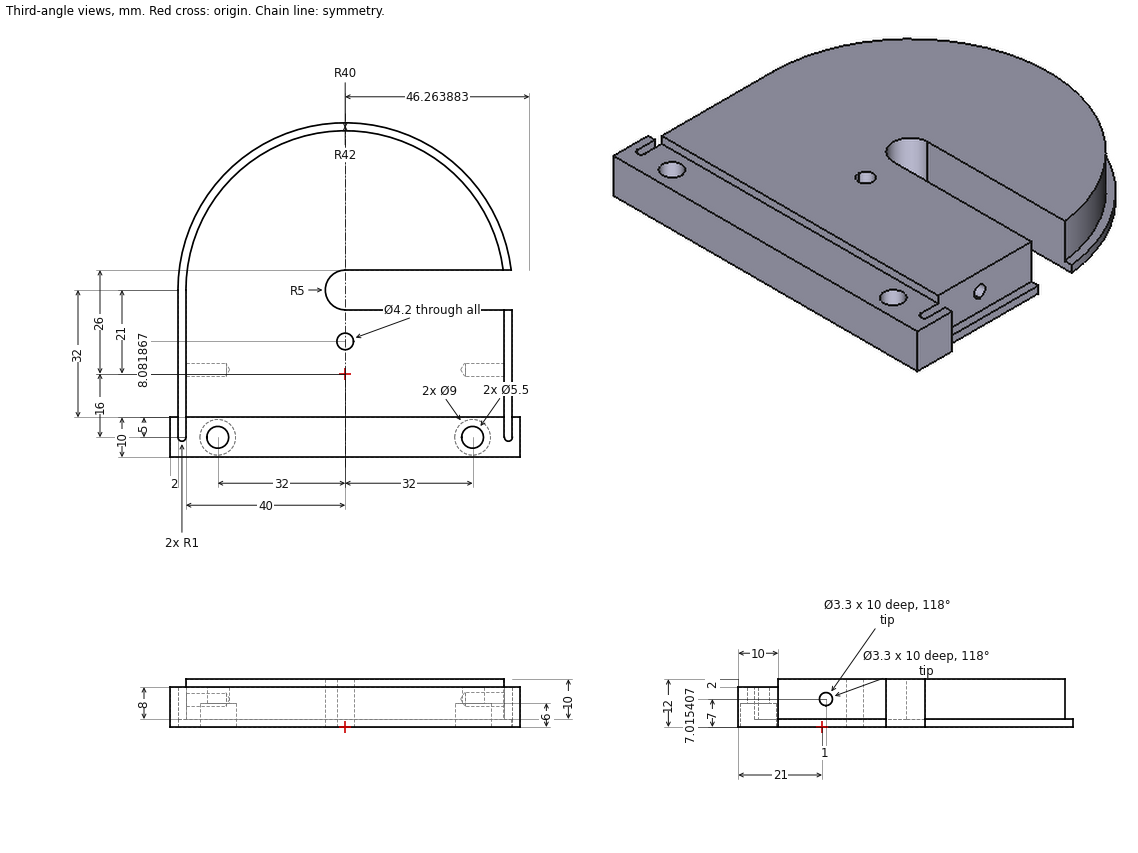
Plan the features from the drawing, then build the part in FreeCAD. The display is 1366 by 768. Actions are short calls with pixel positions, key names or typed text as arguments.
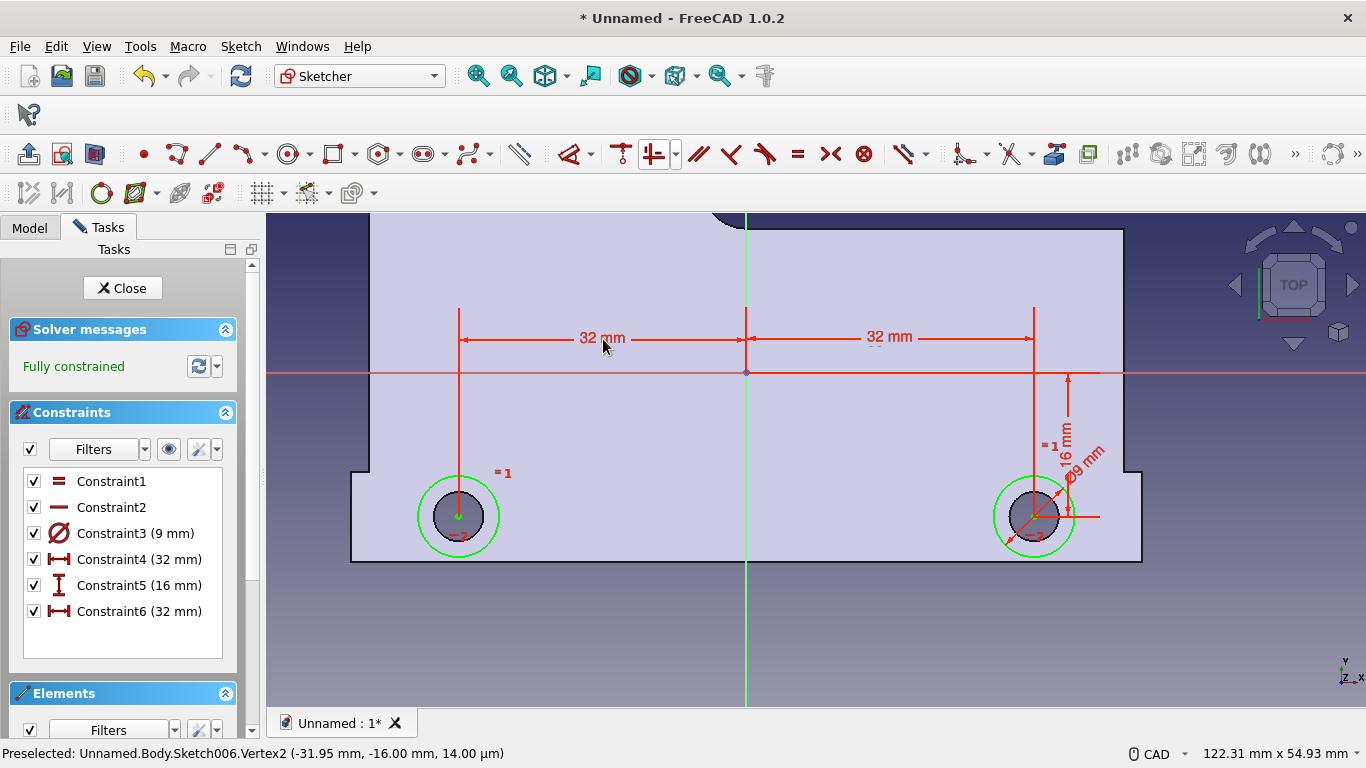
click(123, 288)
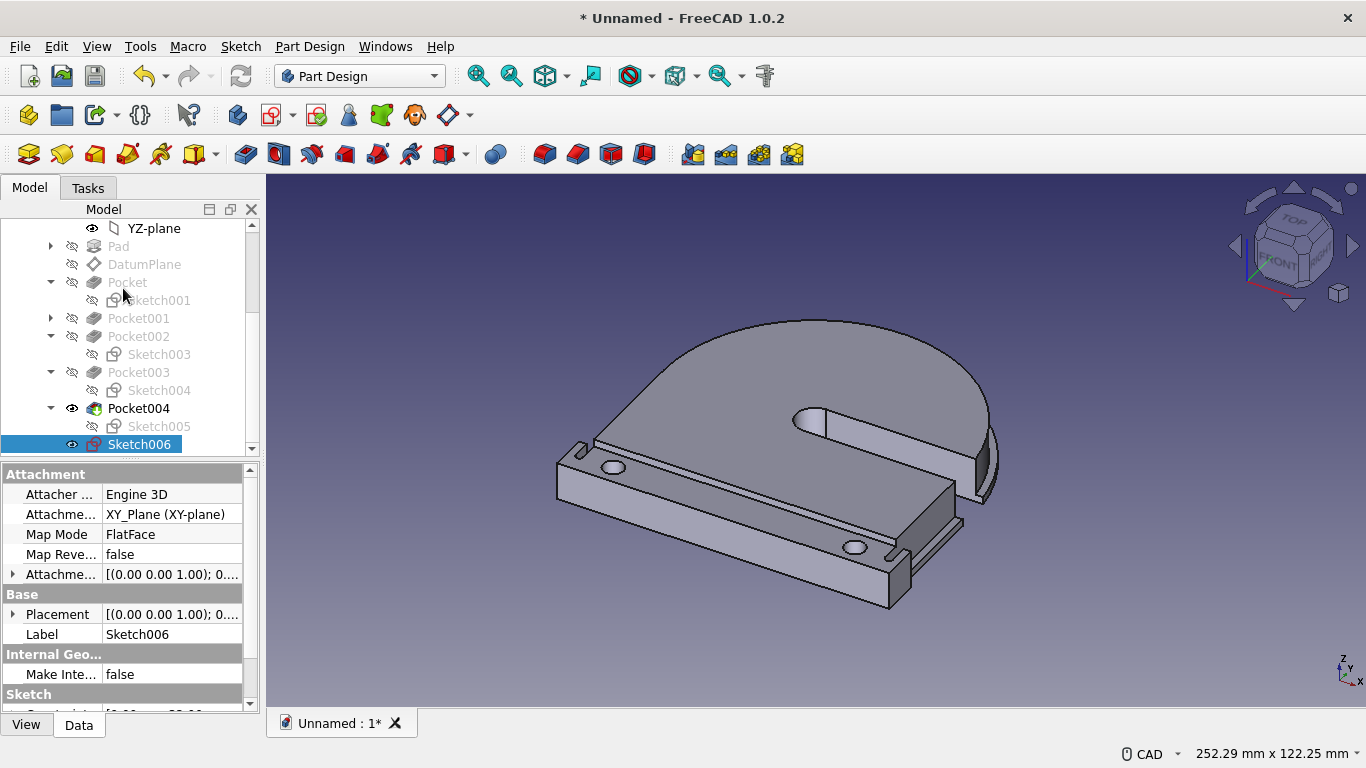
click(246, 154)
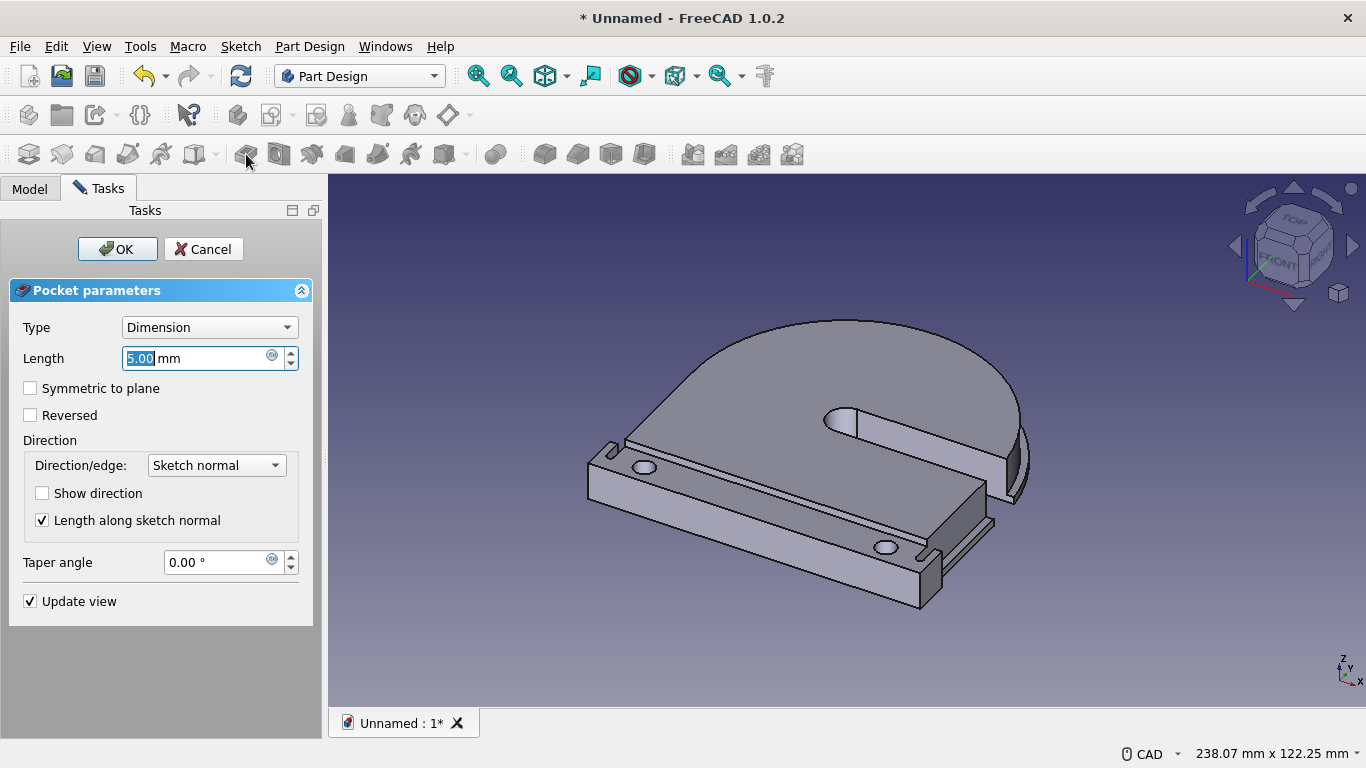
text(6)
key(Tab)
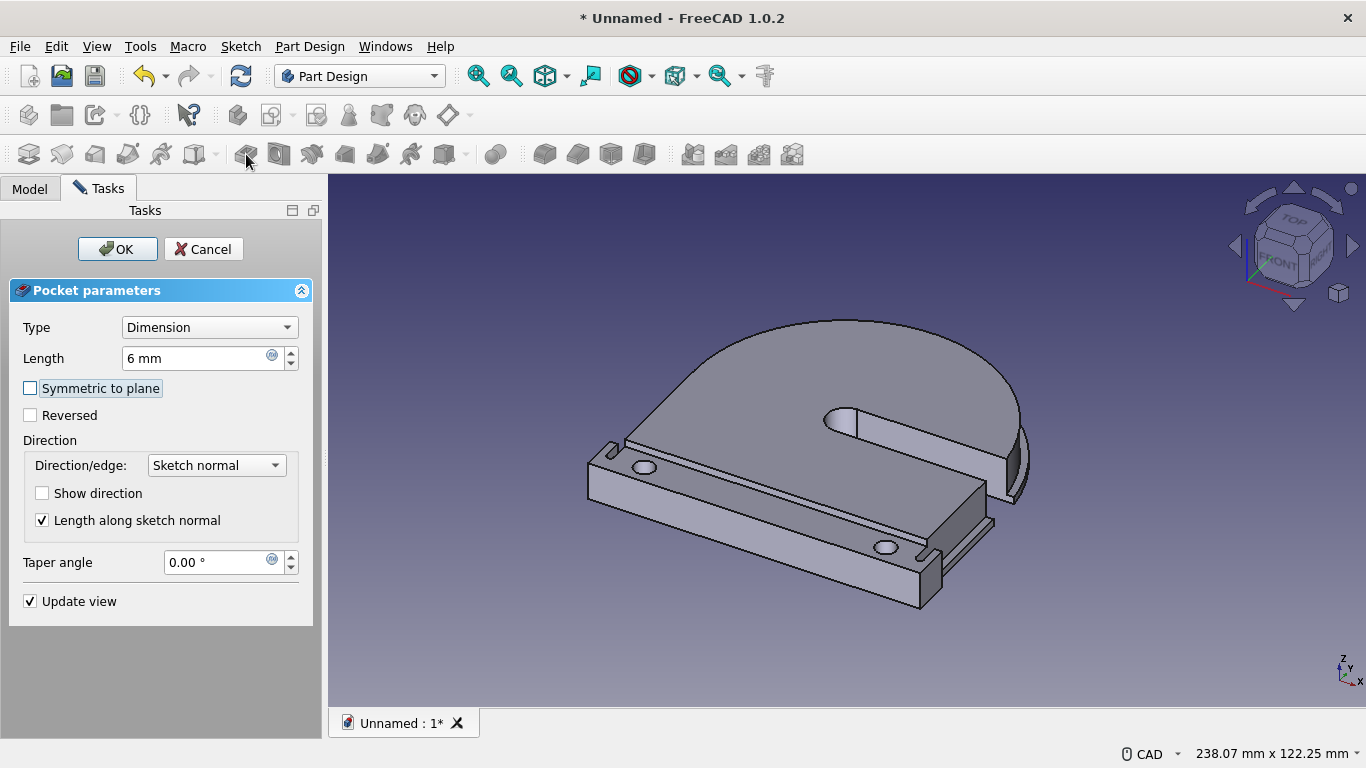
click(31, 415)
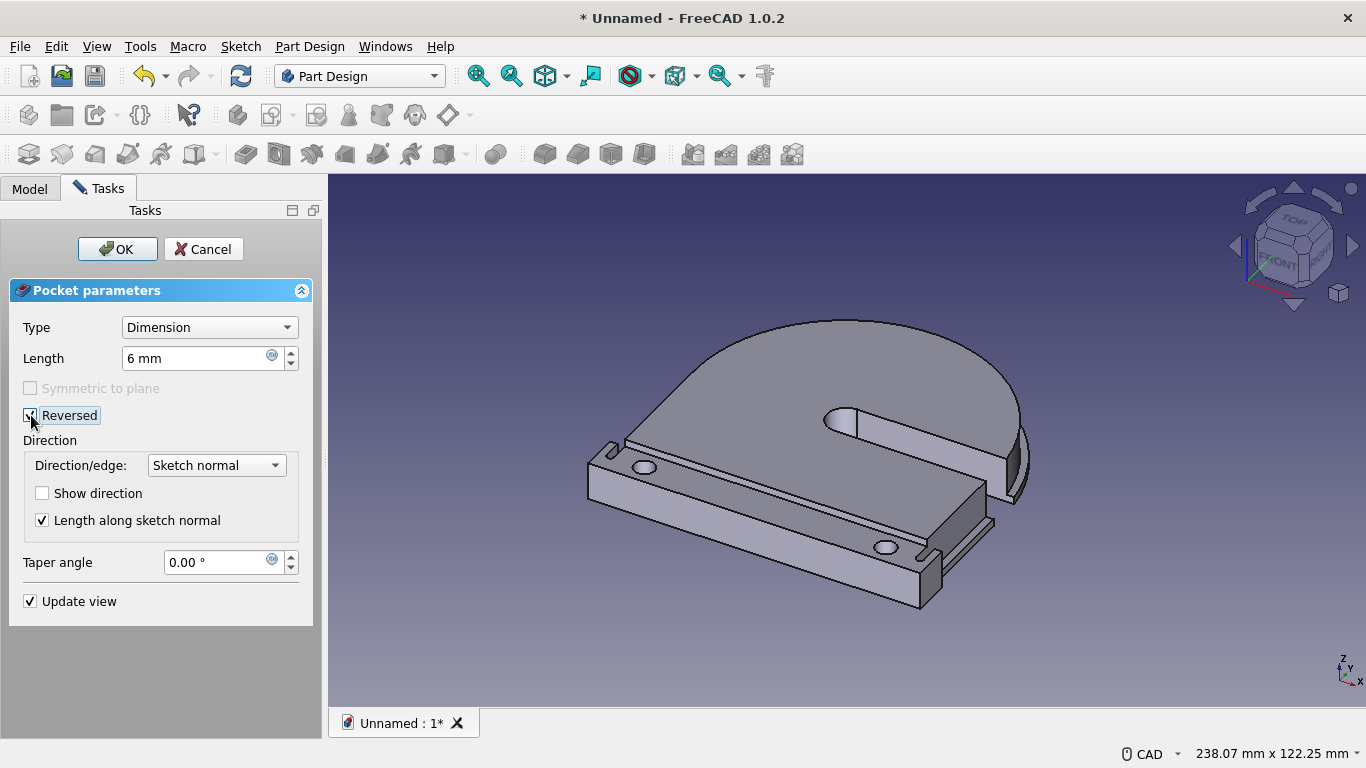
click(118, 249)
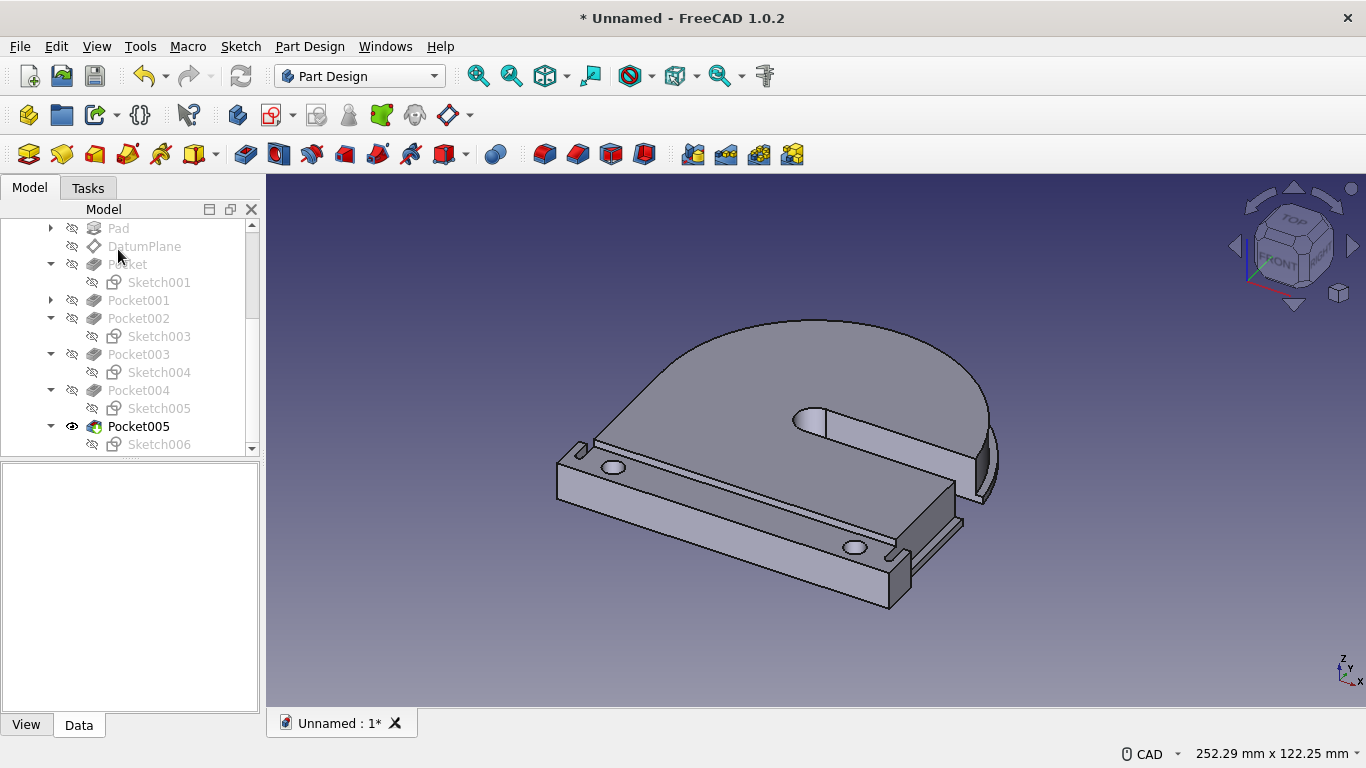
key(6)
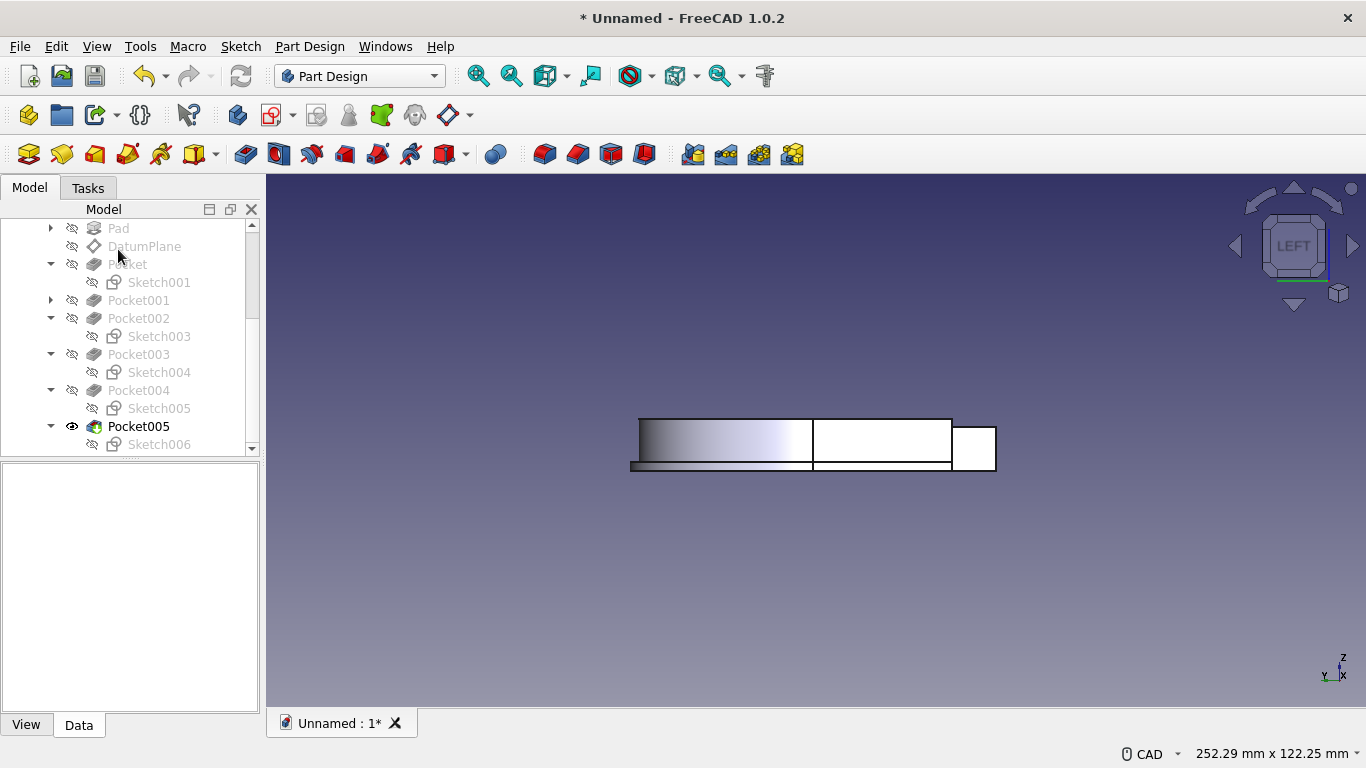
key(v)
key(f)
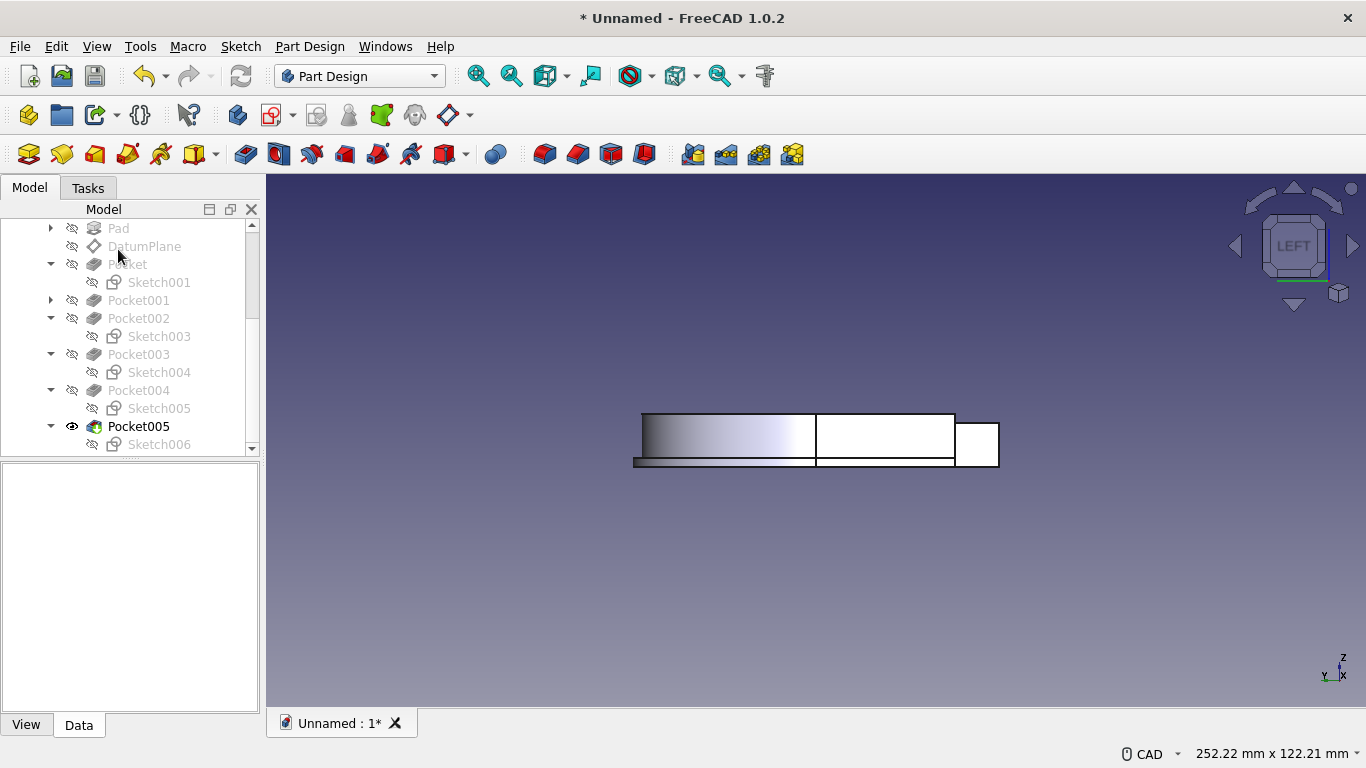
click(850, 435)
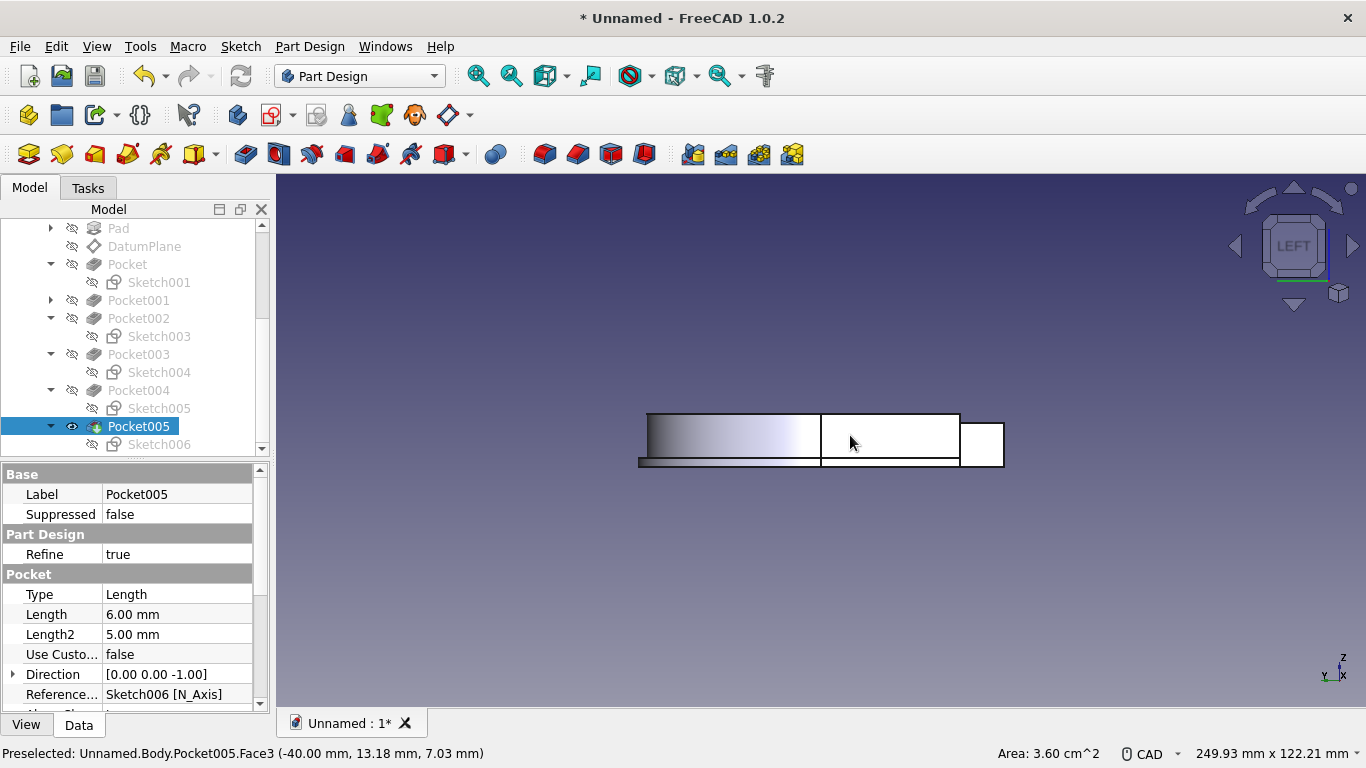
click(270, 116)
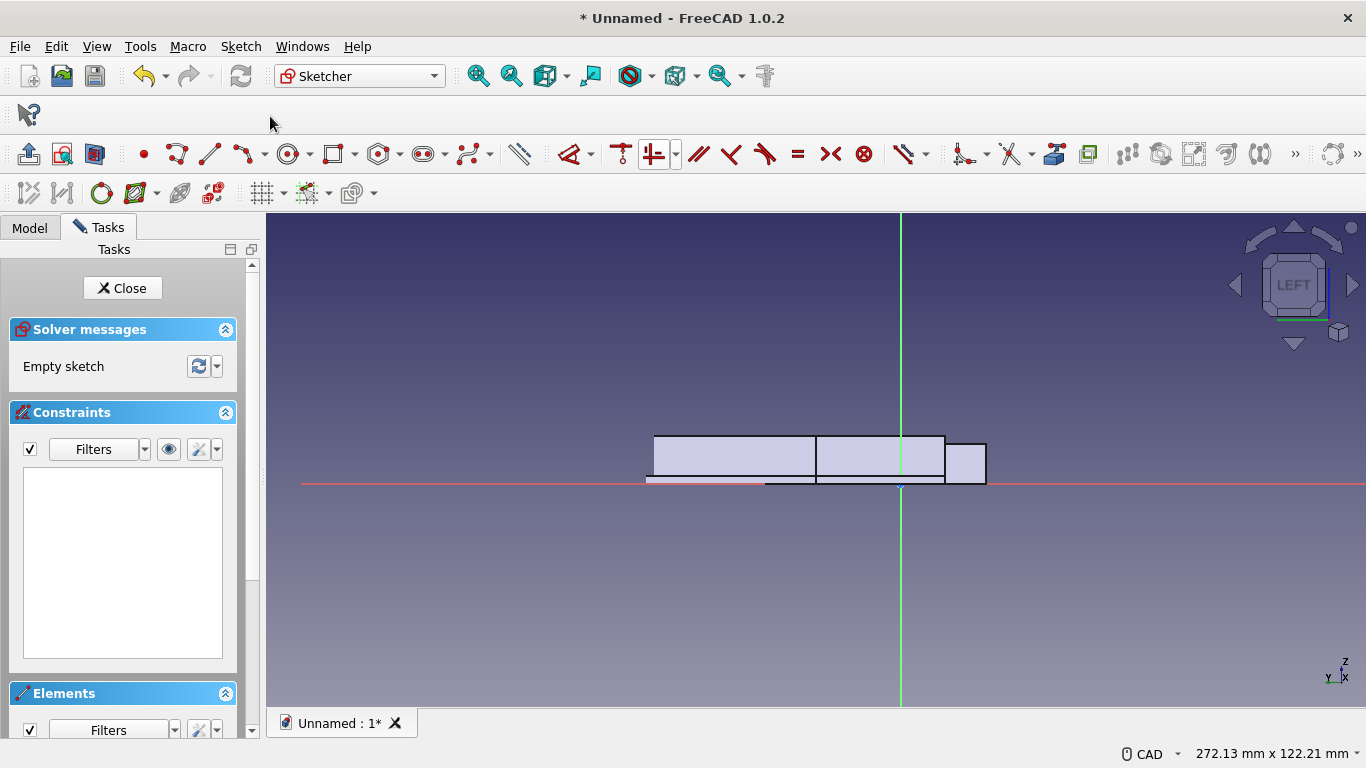
scroll(905, 456, up, 15)